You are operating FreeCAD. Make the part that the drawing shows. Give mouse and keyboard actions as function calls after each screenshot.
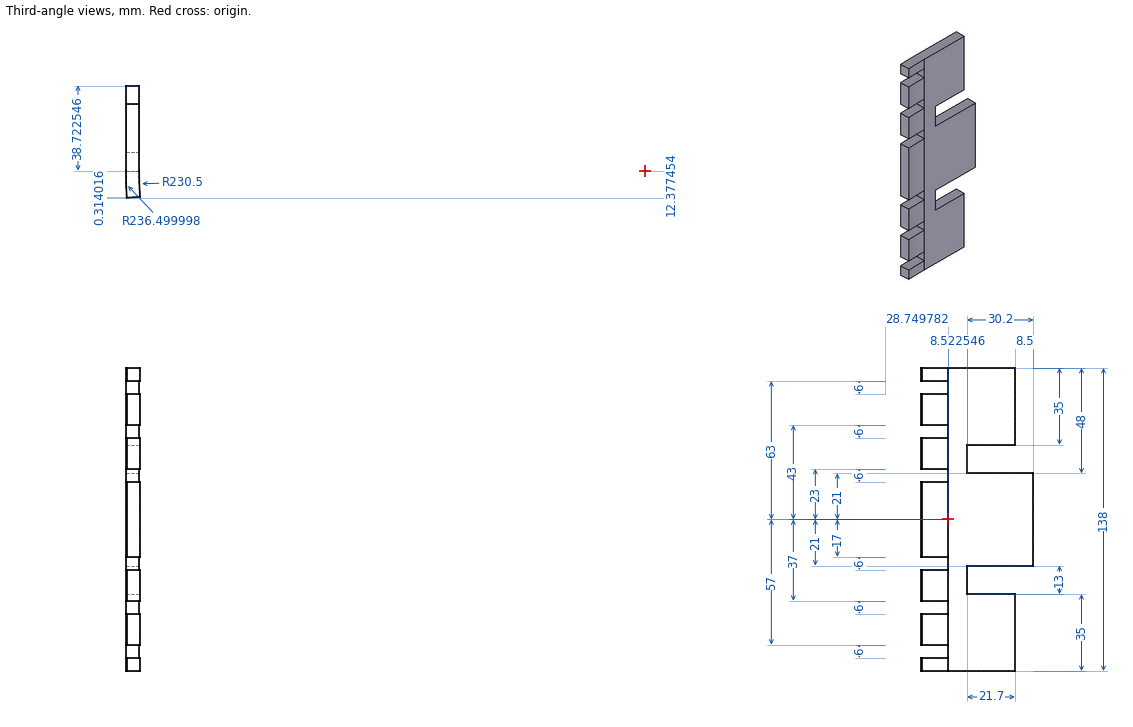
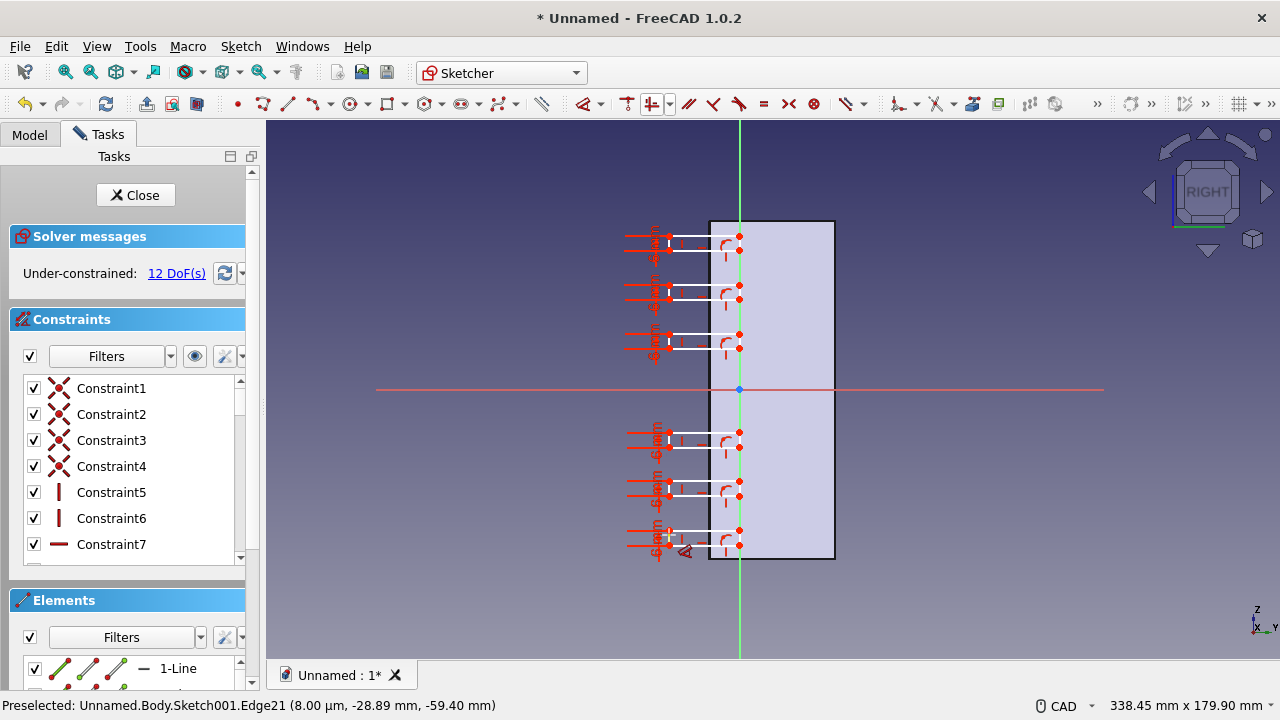
click(669, 236)
click(635, 313)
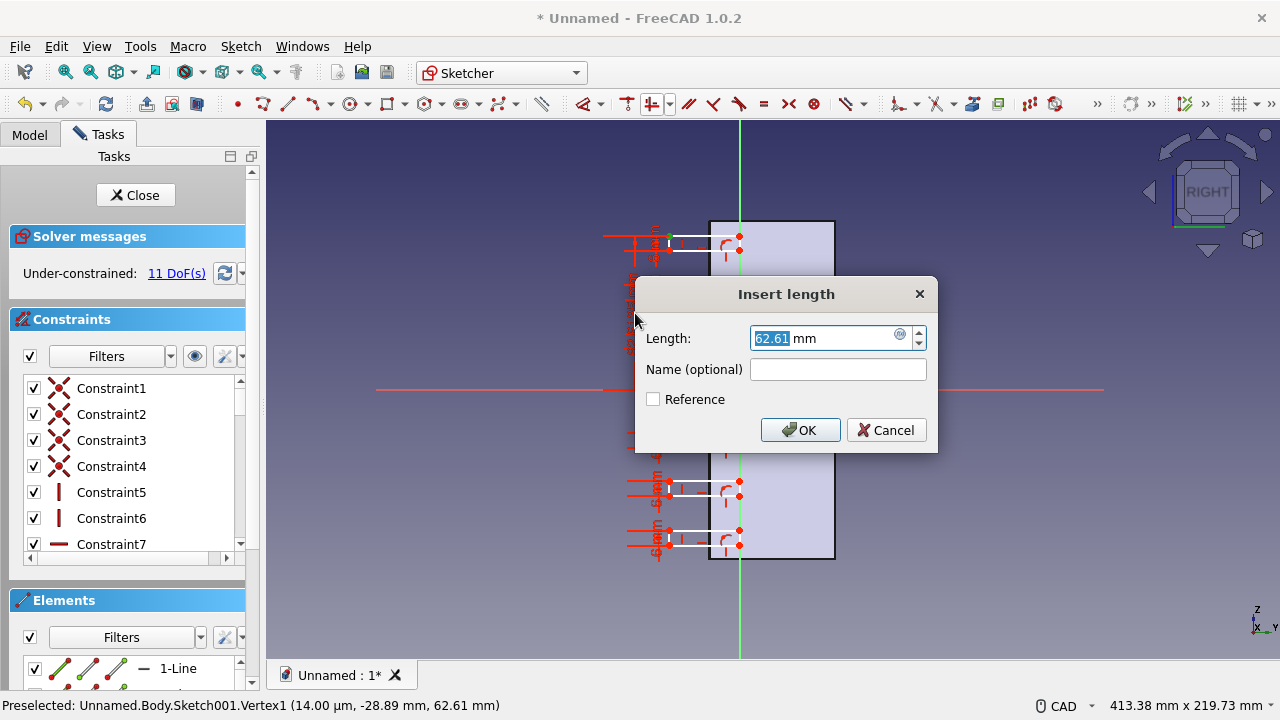
text(63)
key(Return)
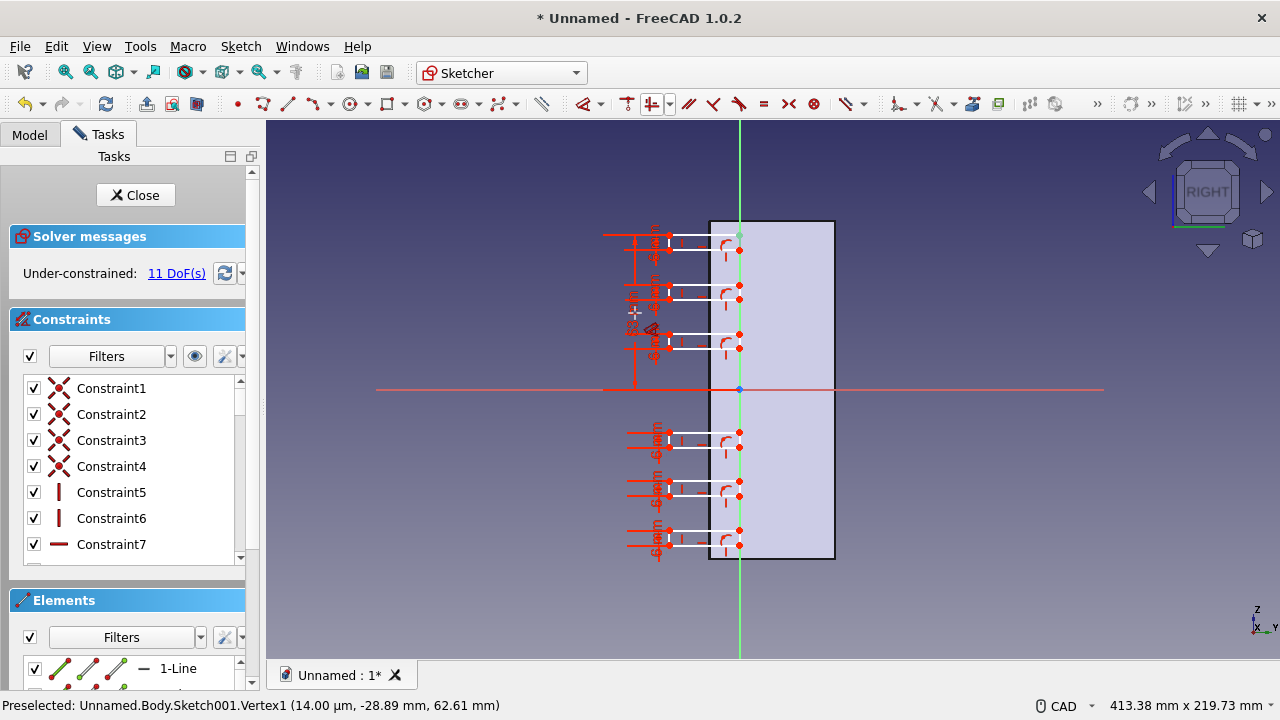
click(669, 285)
click(635, 362)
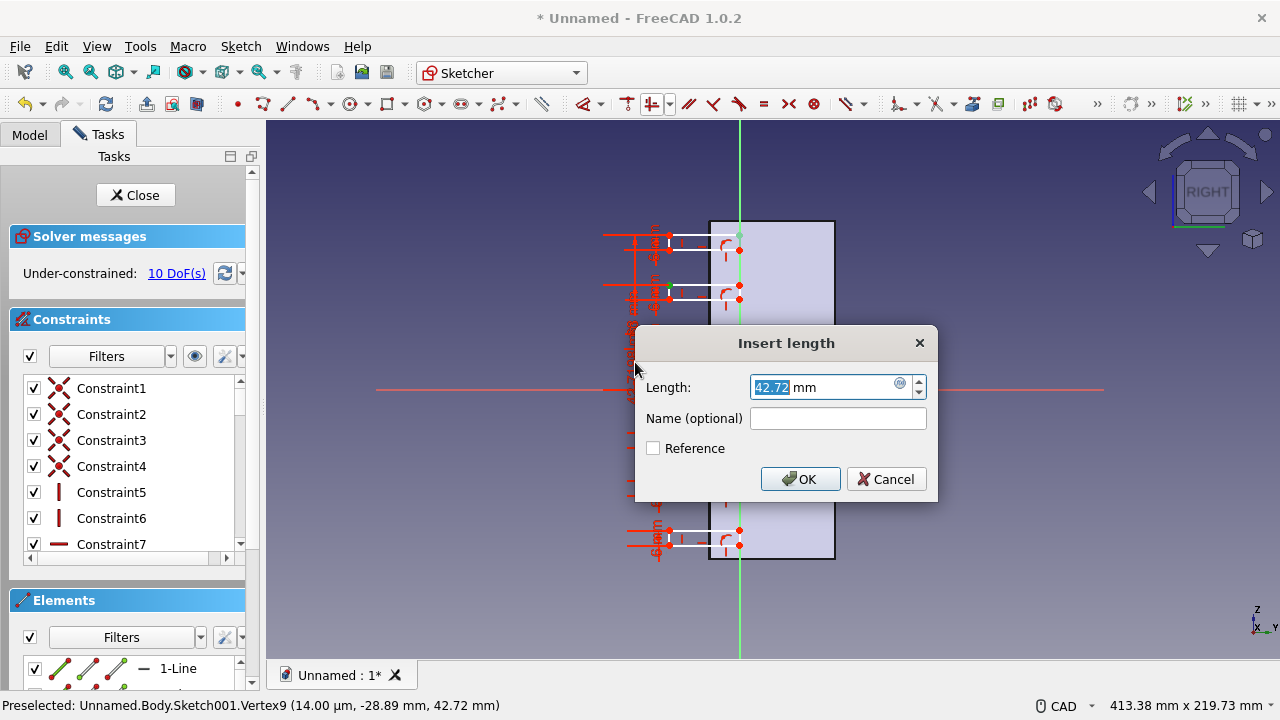
text(43)
key(Return)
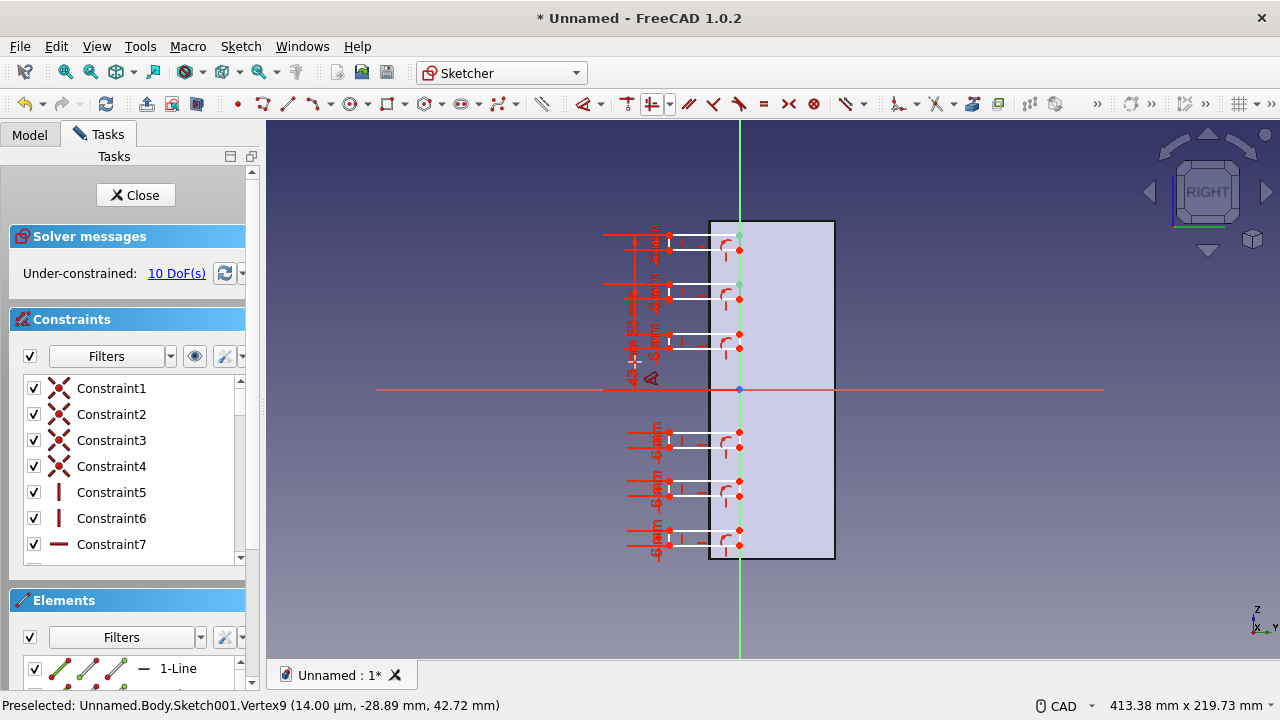
click(669, 334)
click(774, 362)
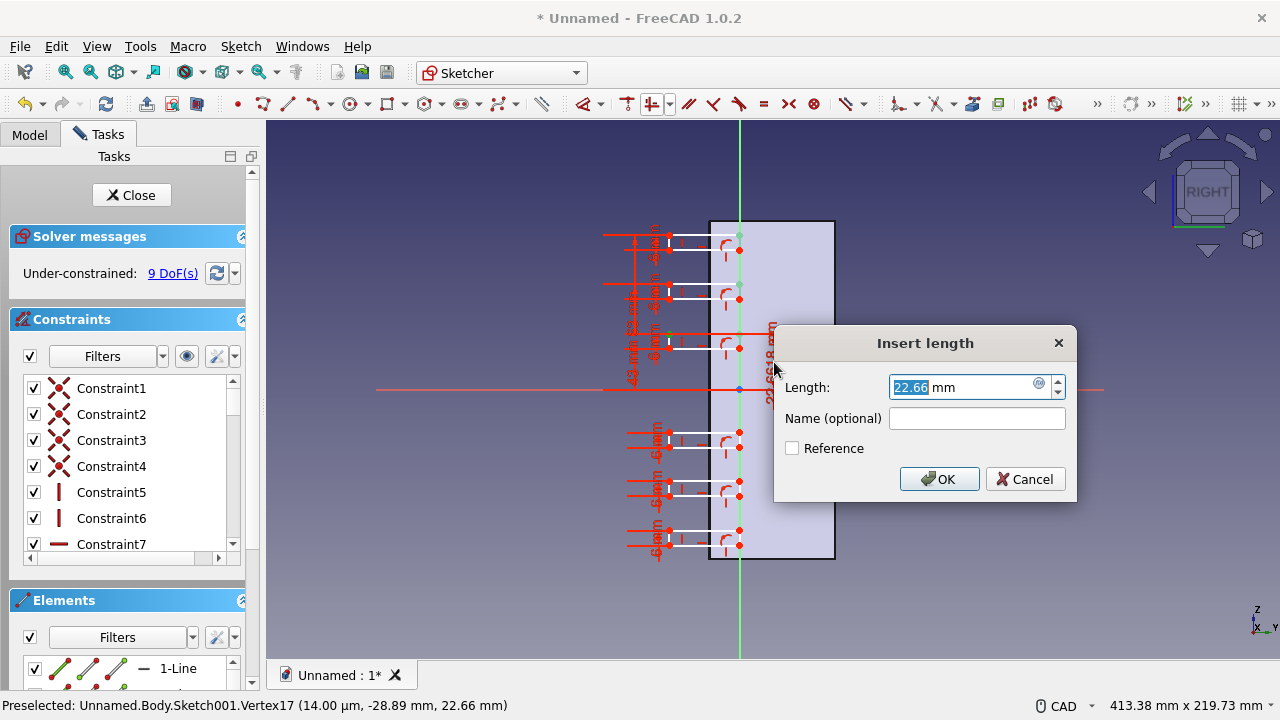
text(23)
key(Return)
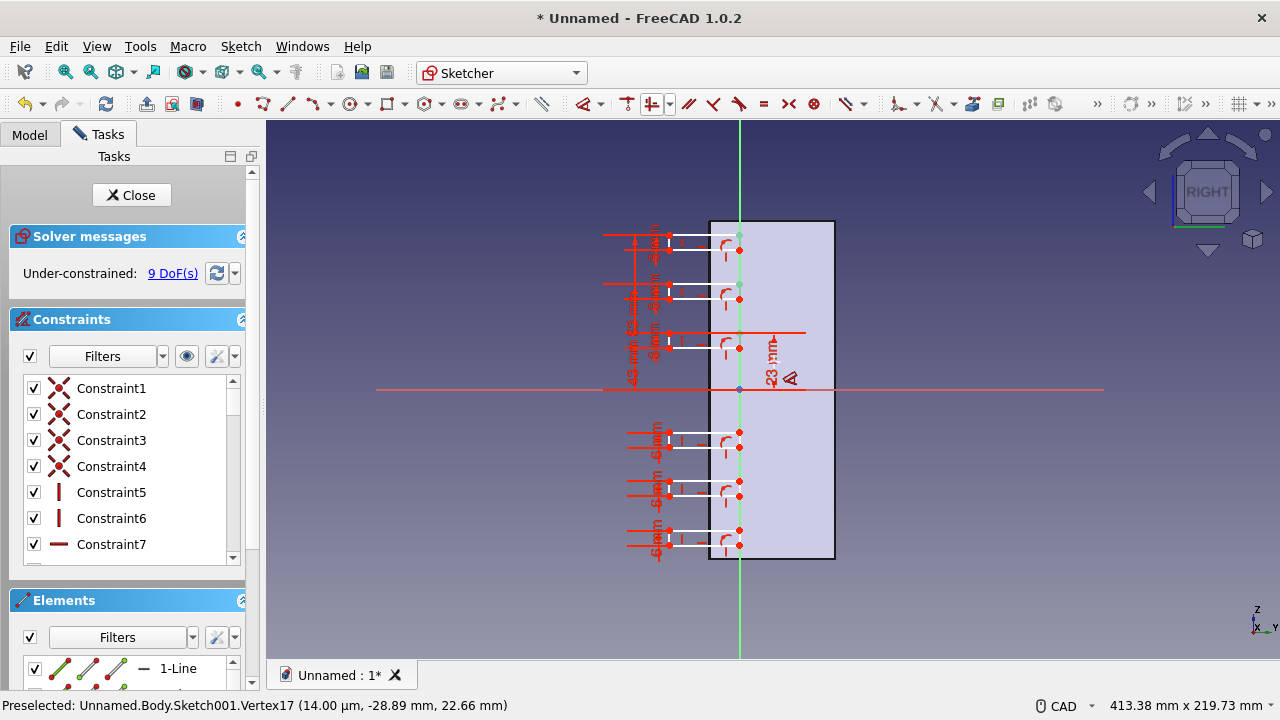
click(669, 433)
click(635, 411)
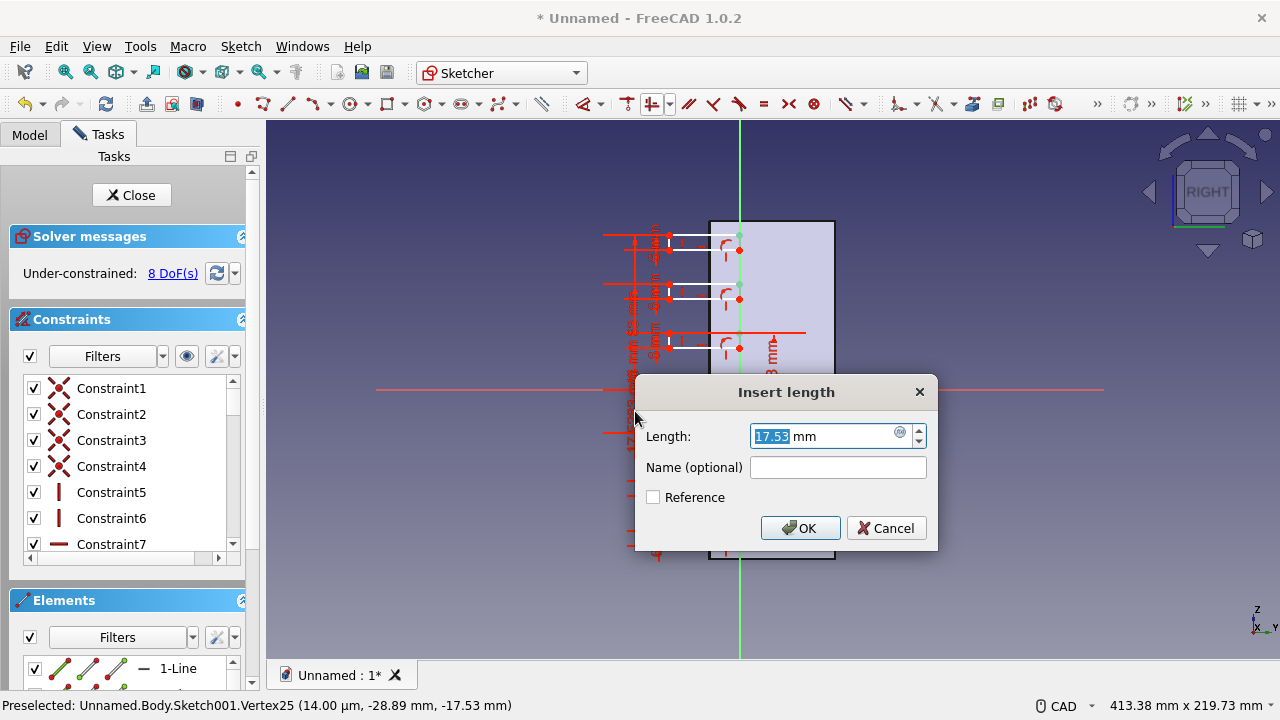
text(17)
key(Return)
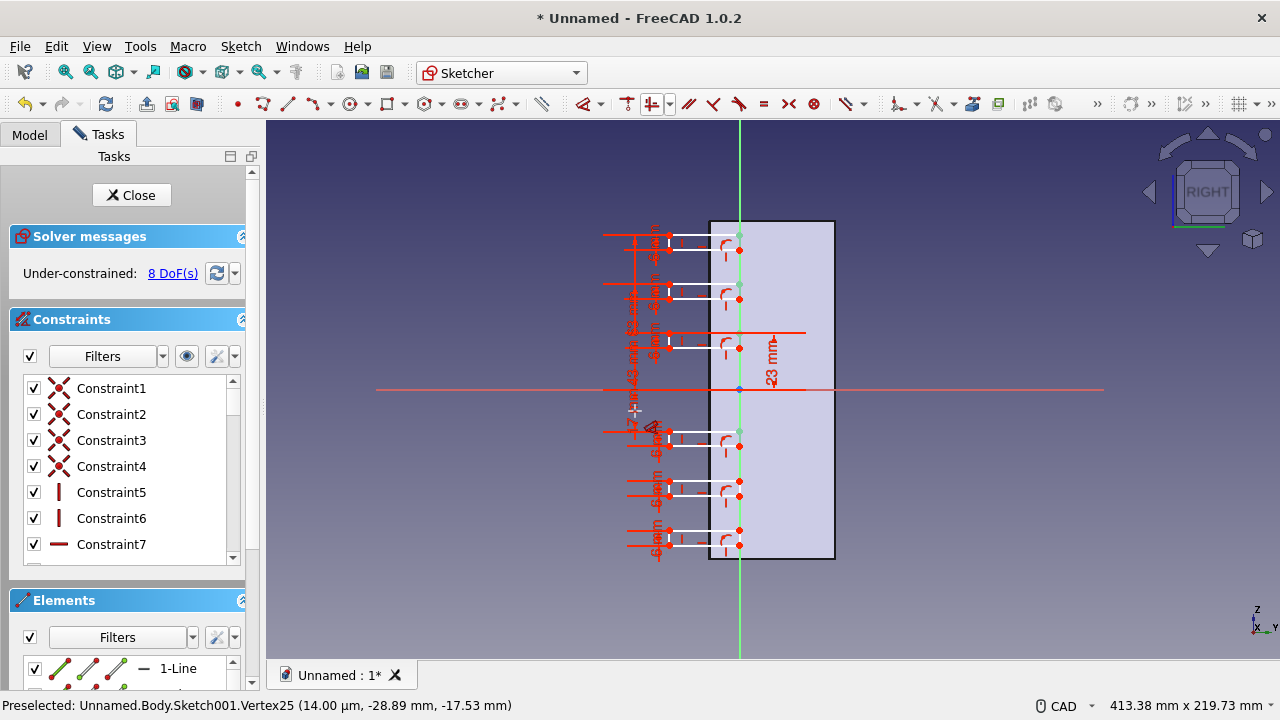
click(669, 481)
click(635, 468)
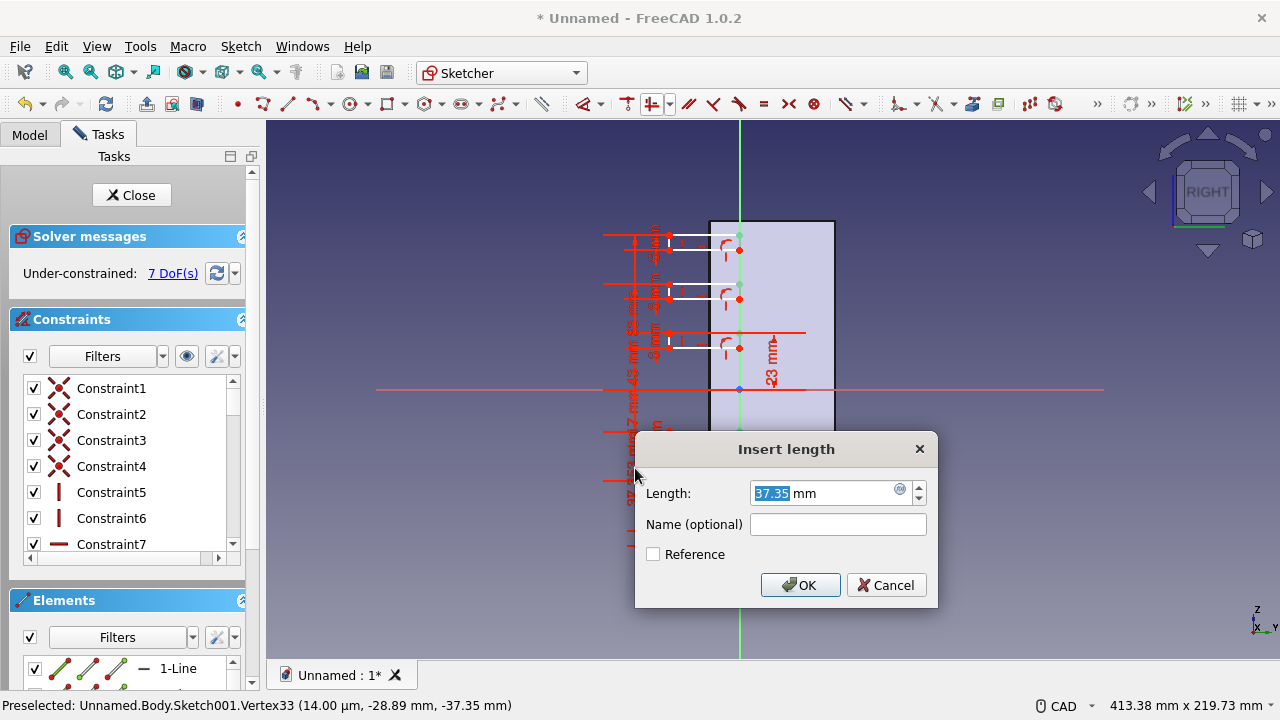
text(37)
key(Return)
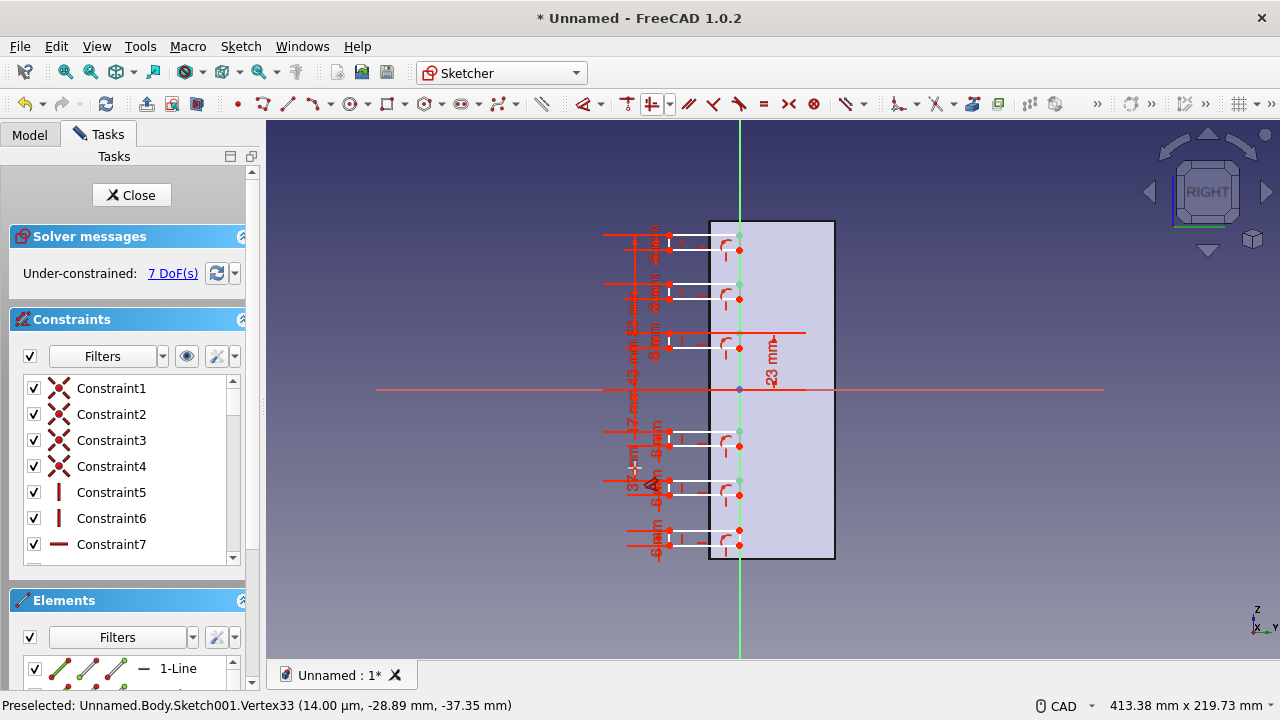
click(669, 531)
click(635, 510)